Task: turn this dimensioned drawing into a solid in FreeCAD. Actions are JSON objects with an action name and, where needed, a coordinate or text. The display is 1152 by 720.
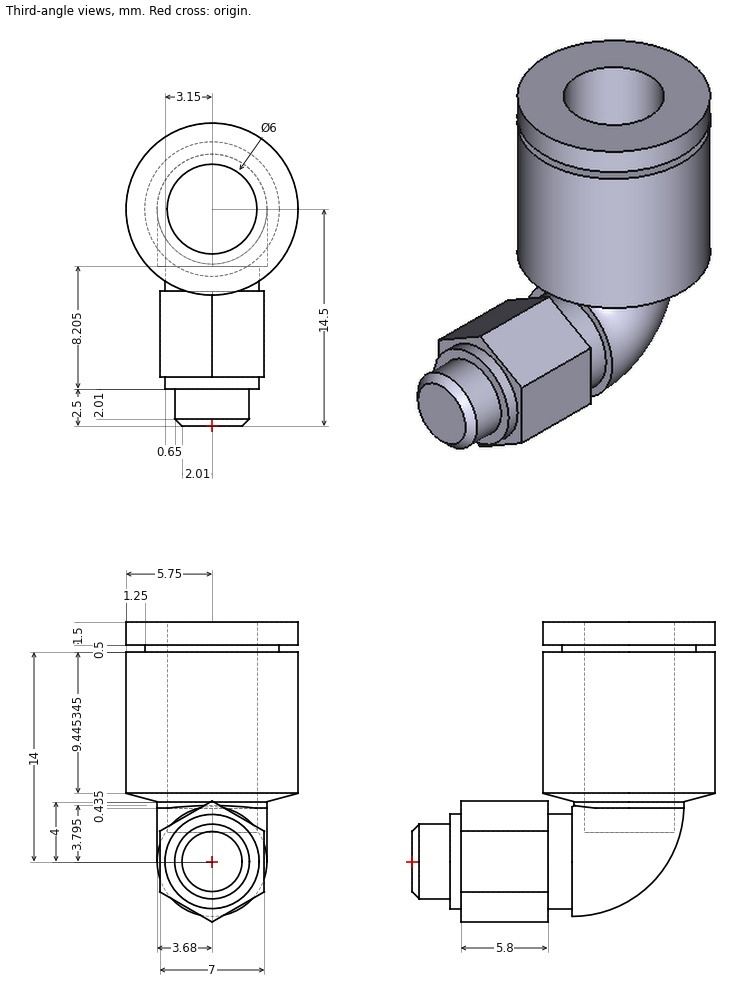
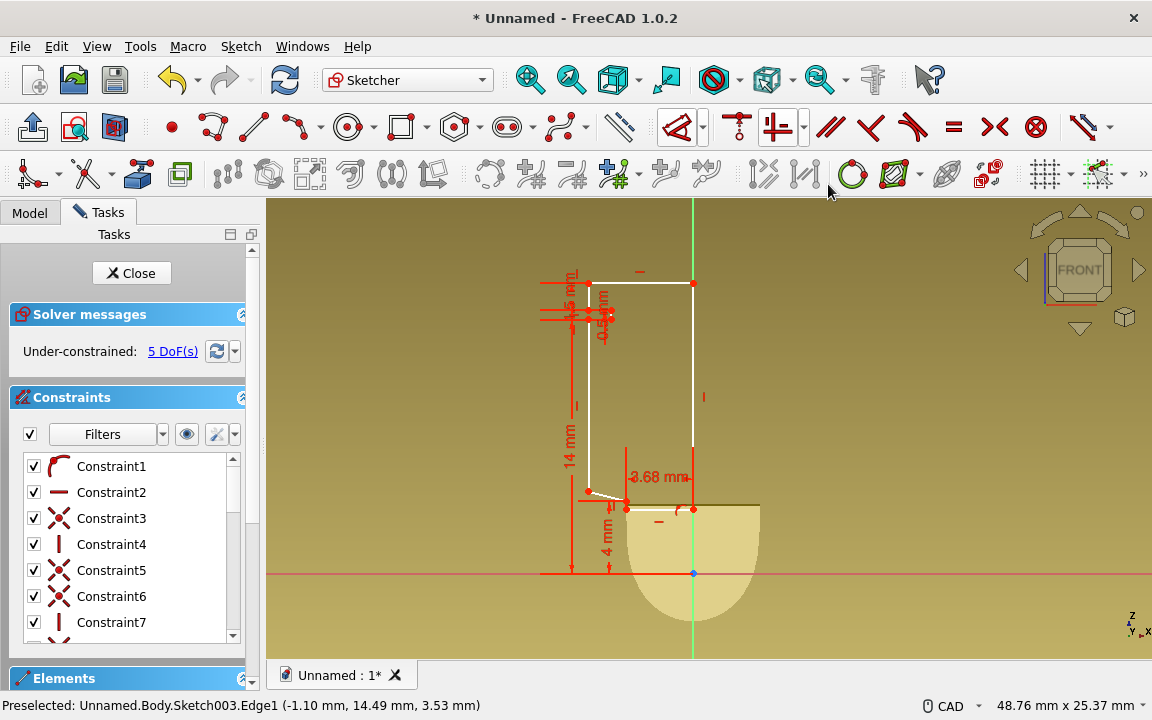
{"action": "scroll", "coordinate": [600, 320], "scroll_direction": "up", "scroll_amount": 3}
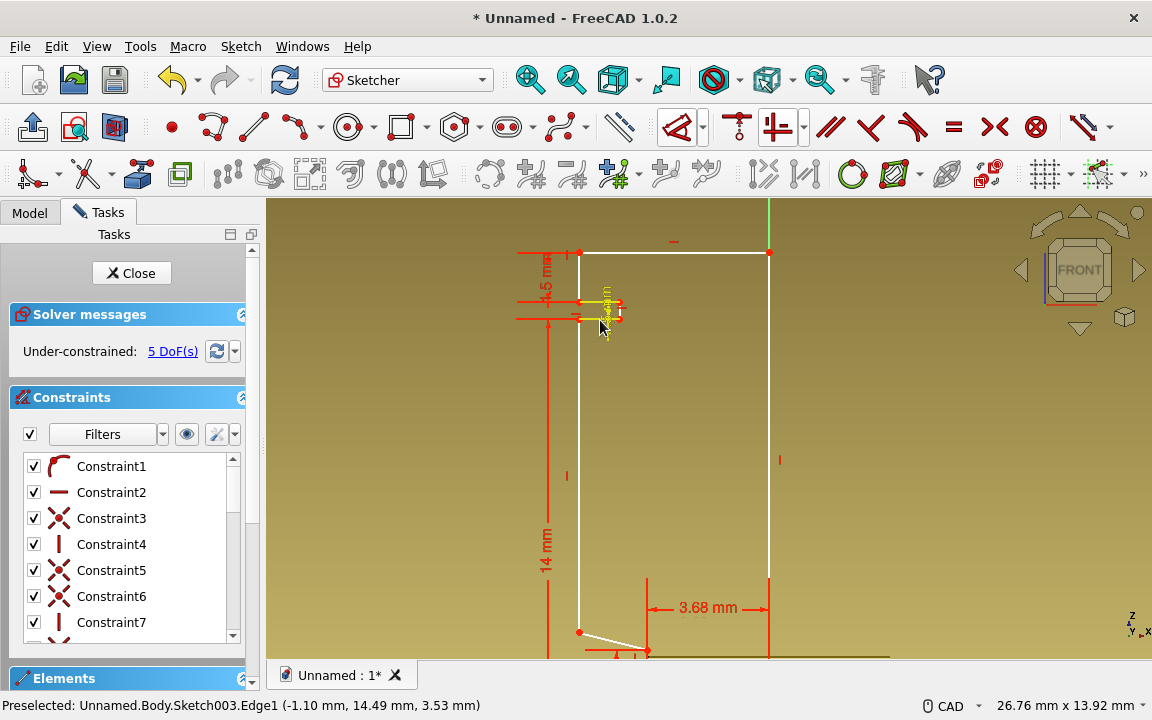
{"action": "left_click", "coordinate": [599, 319]}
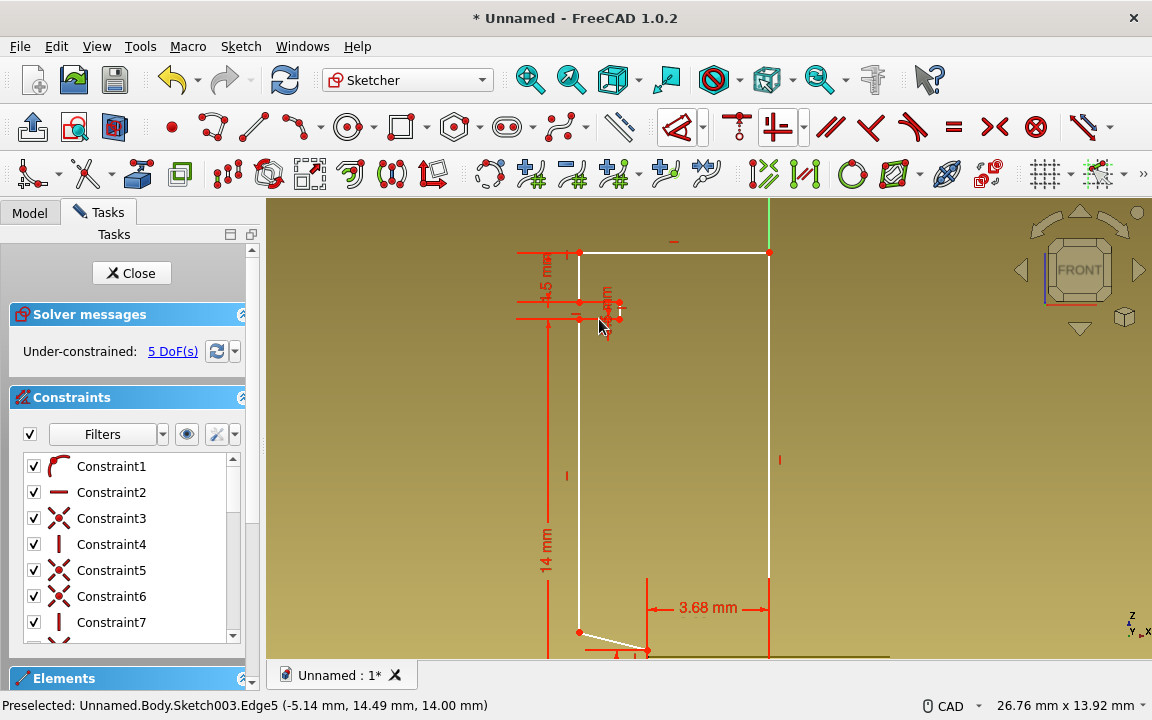
{"action": "left_click", "coordinate": [702, 128]}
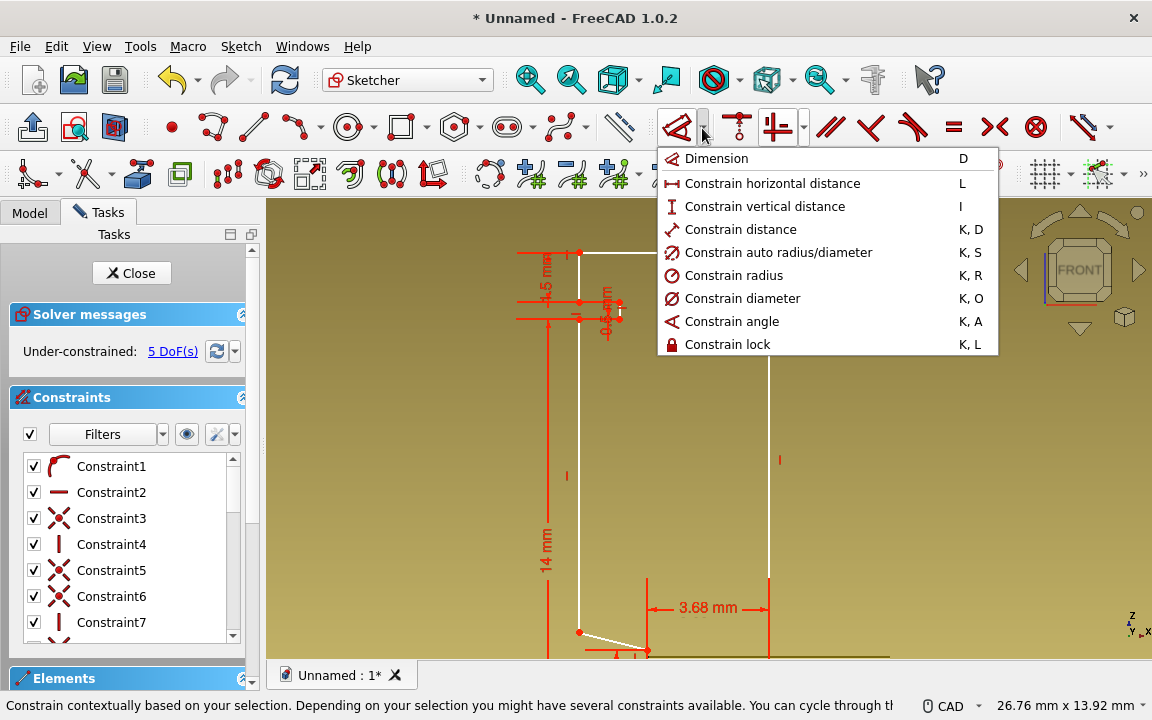
{"action": "left_click", "coordinate": [828, 184]}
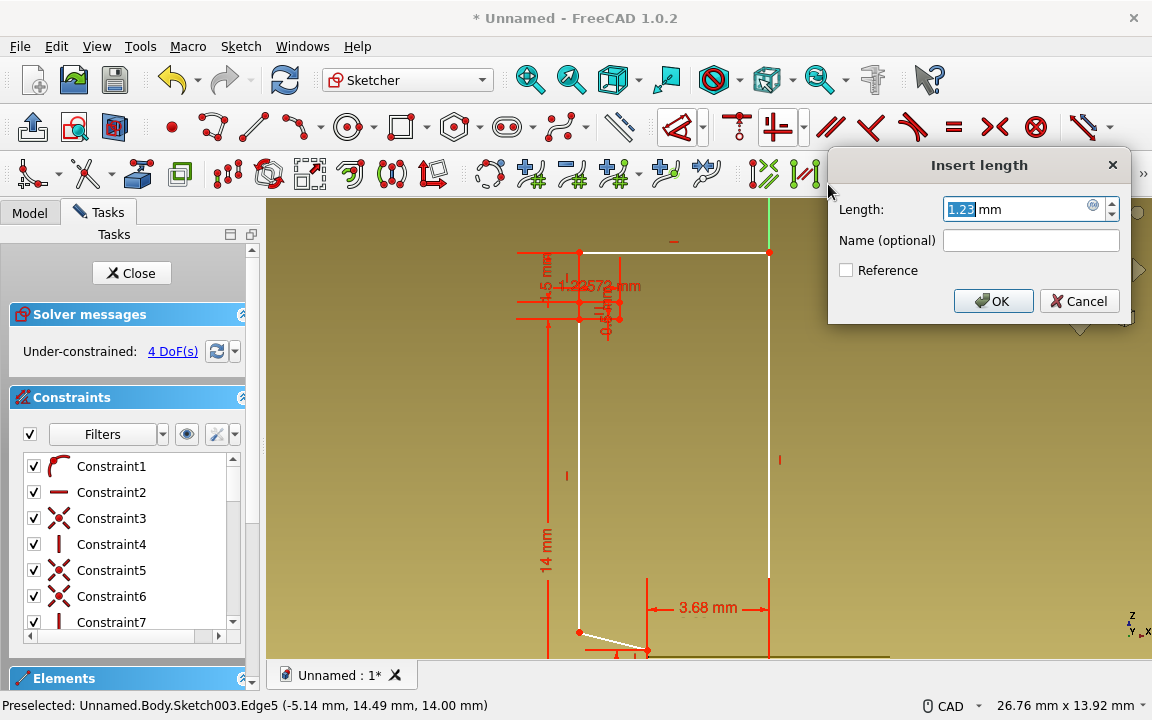
{"action": "type", "text": "1.25"}
{"action": "key", "text": "Return"}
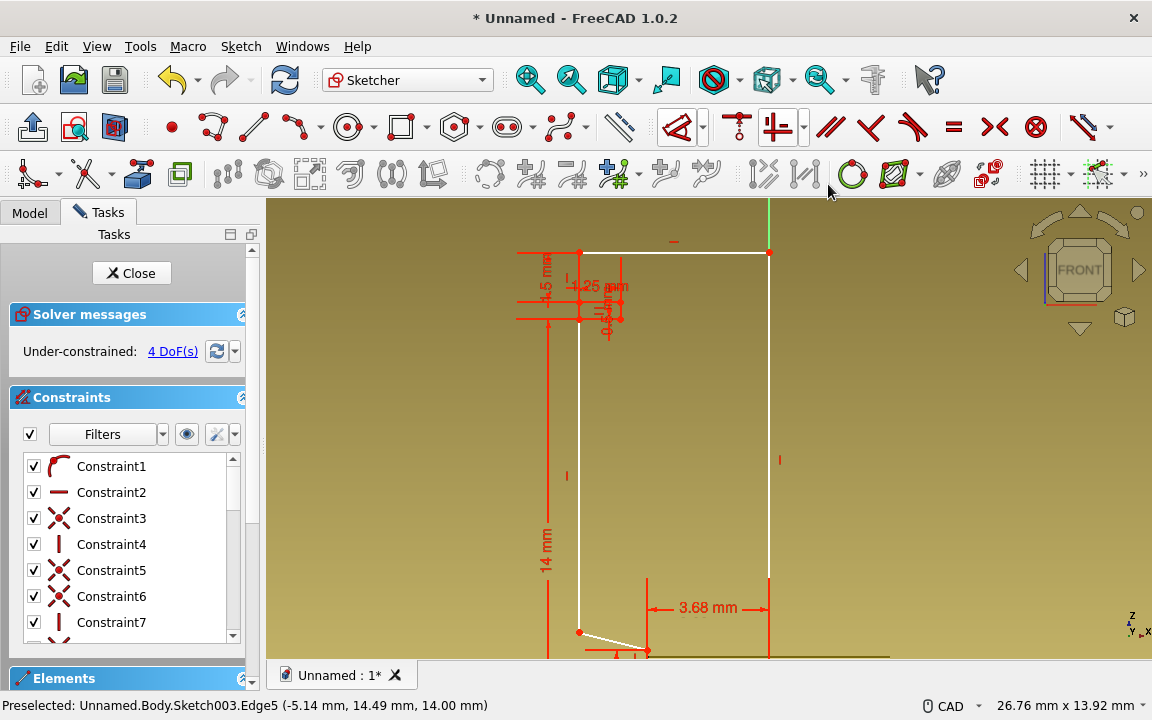
{"action": "left_click", "coordinate": [591, 302]}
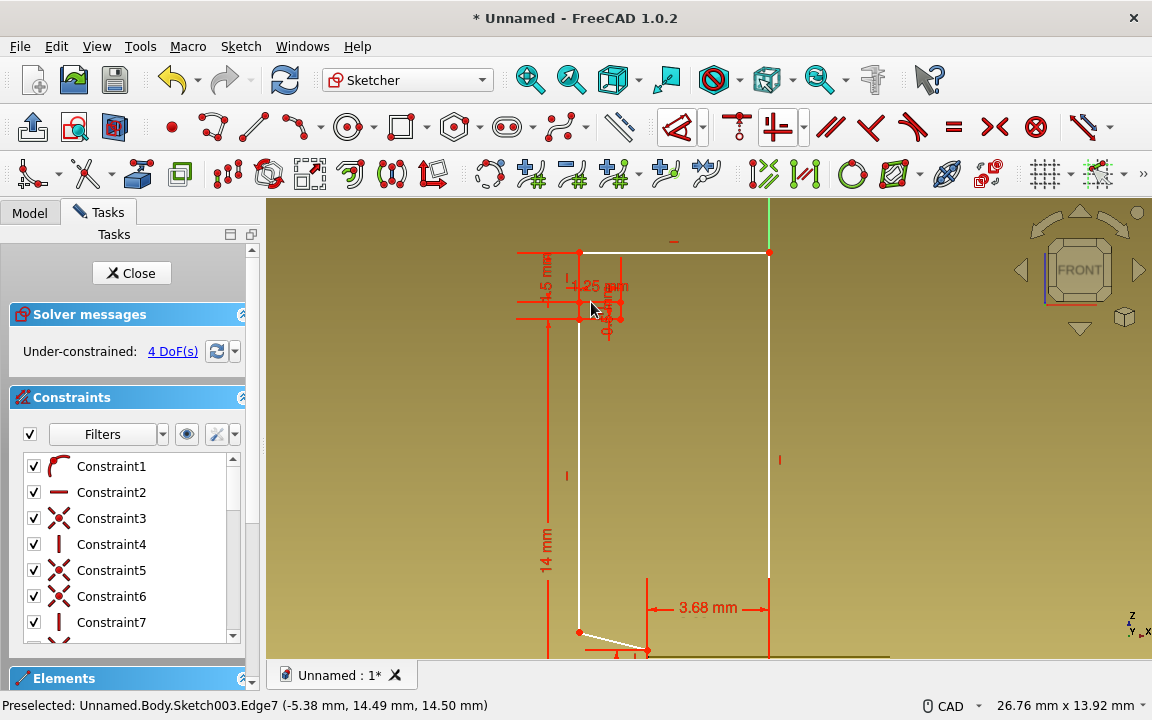
{"action": "left_click", "coordinate": [702, 128]}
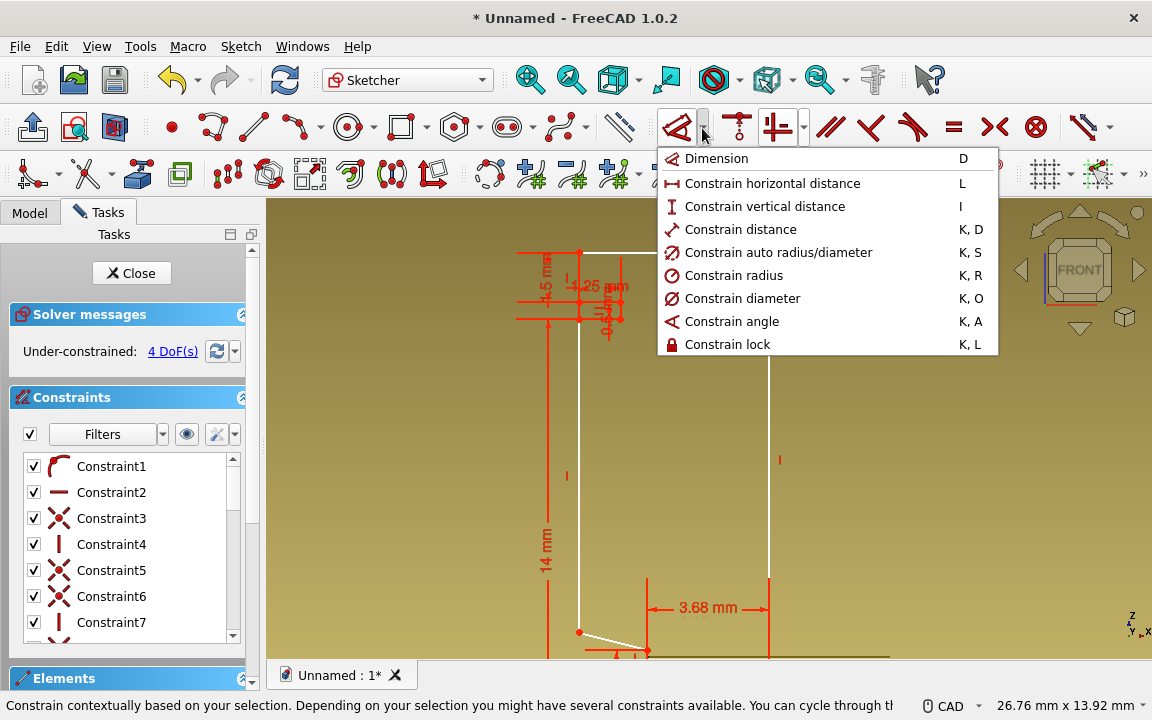
{"action": "left_click", "coordinate": [828, 184]}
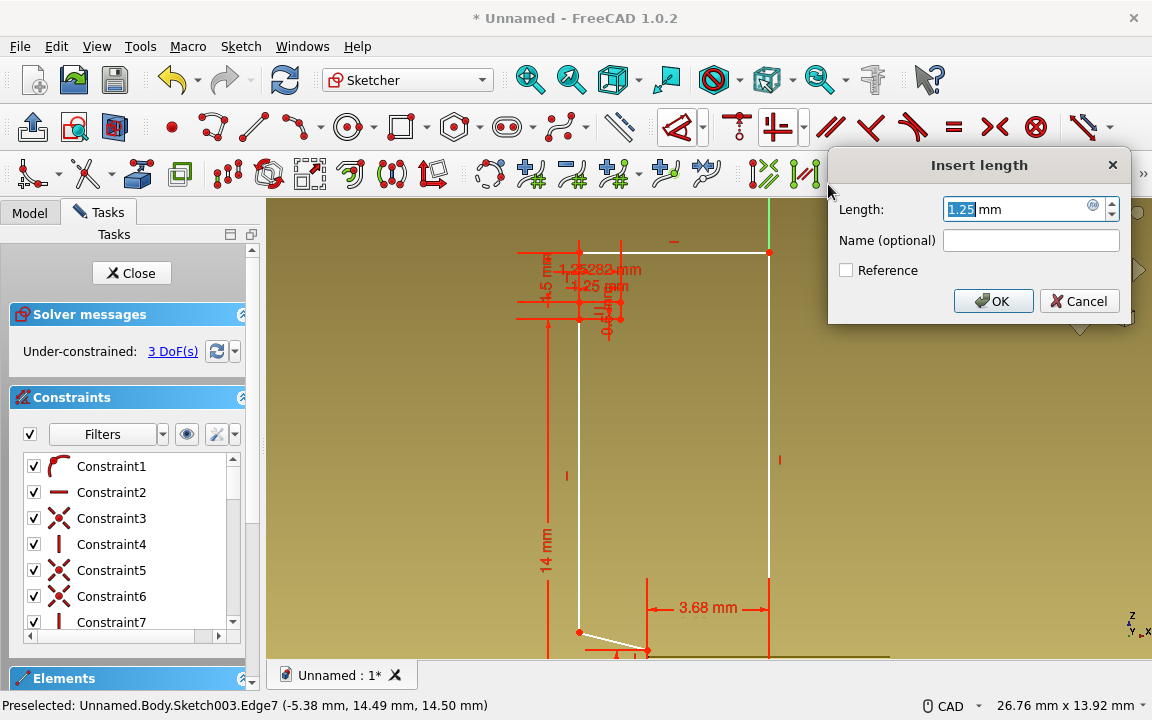
{"action": "type", "text": "1.25"}
{"action": "key", "text": "Return"}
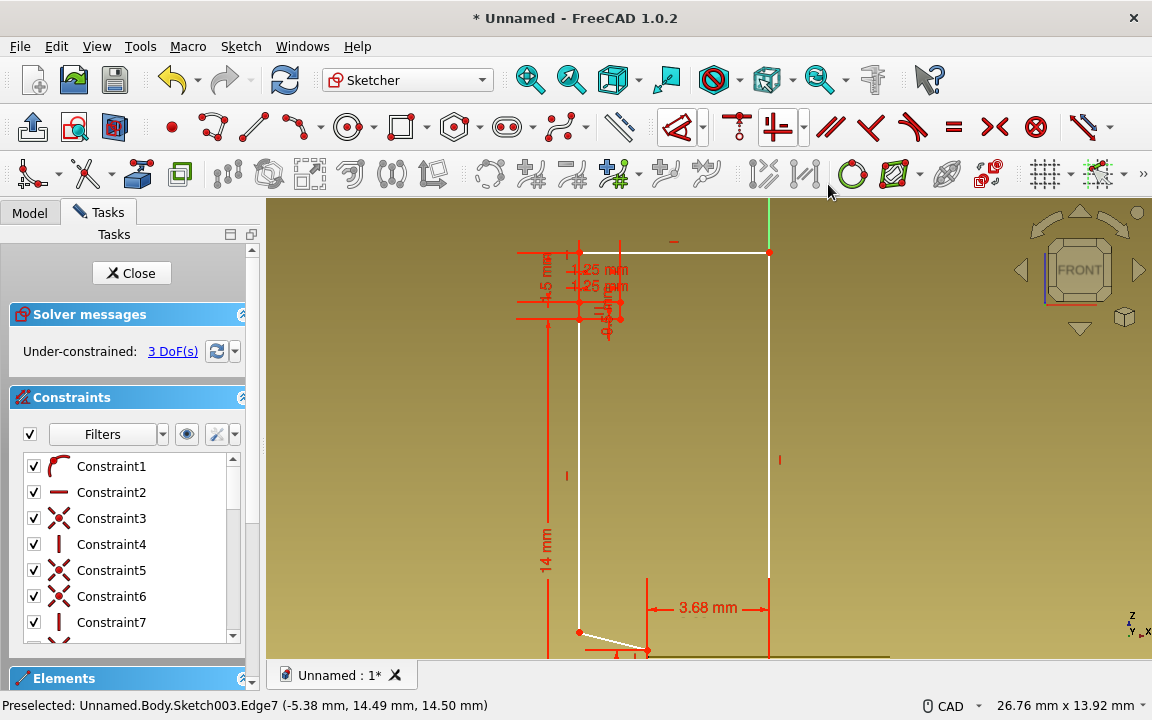
{"action": "left_click", "coordinate": [636, 253]}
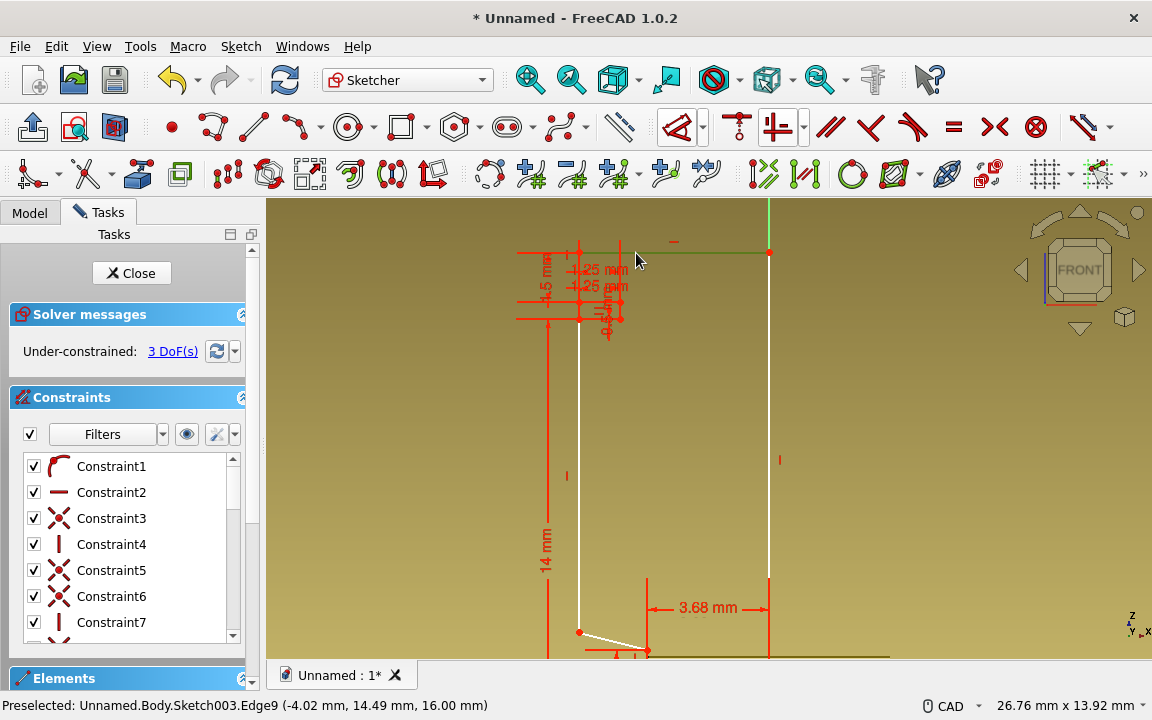
{"action": "key", "text": "l"}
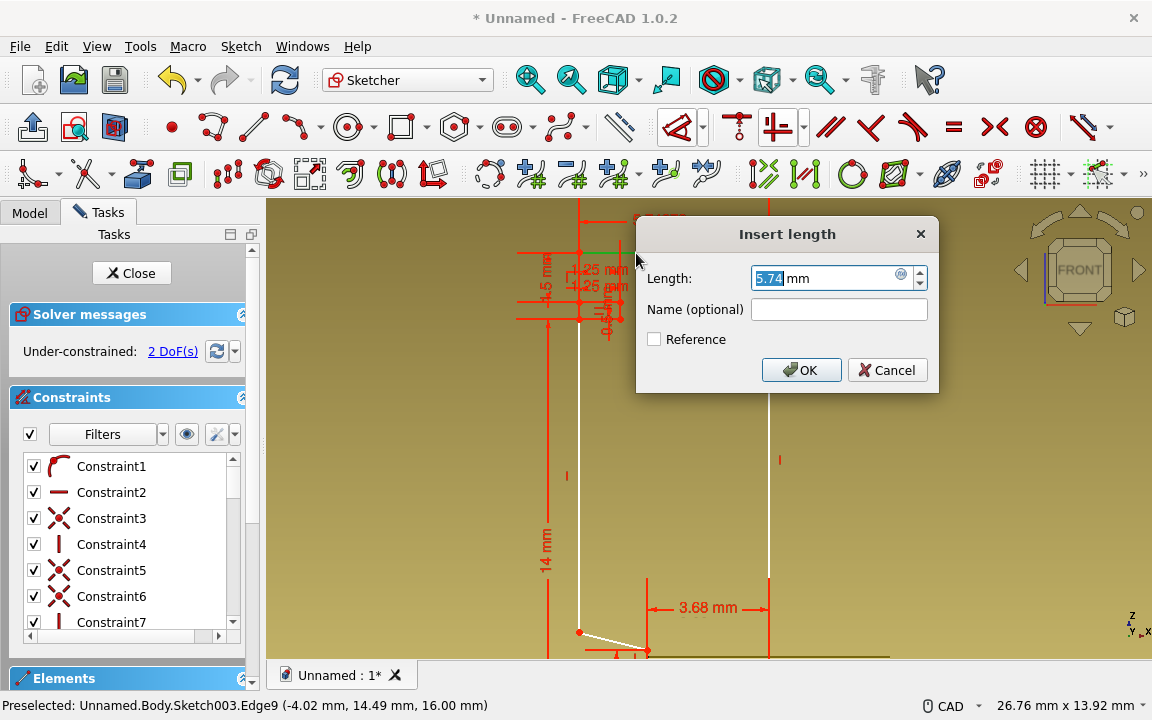
{"action": "type", "text": "5.75"}
{"action": "key", "text": "Return"}